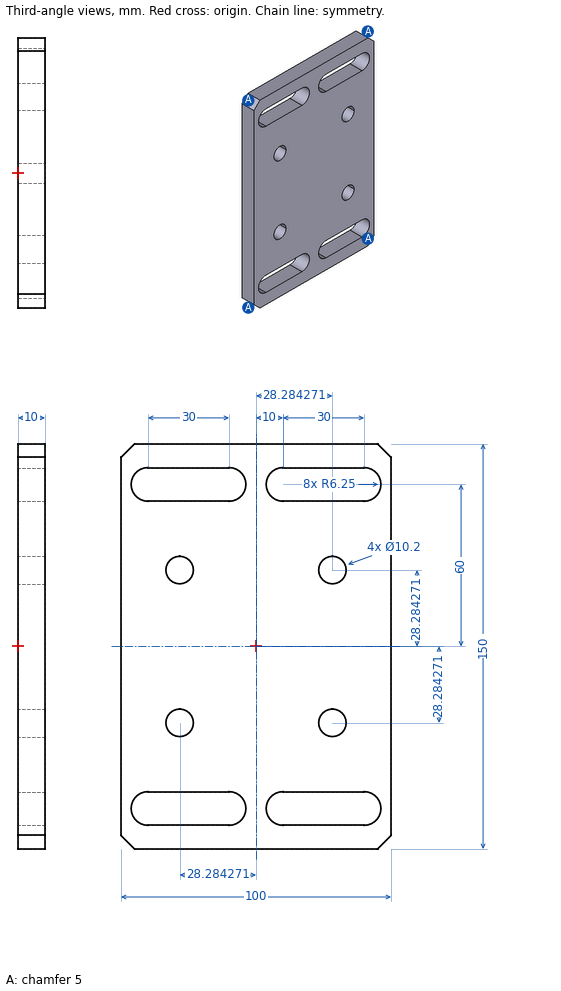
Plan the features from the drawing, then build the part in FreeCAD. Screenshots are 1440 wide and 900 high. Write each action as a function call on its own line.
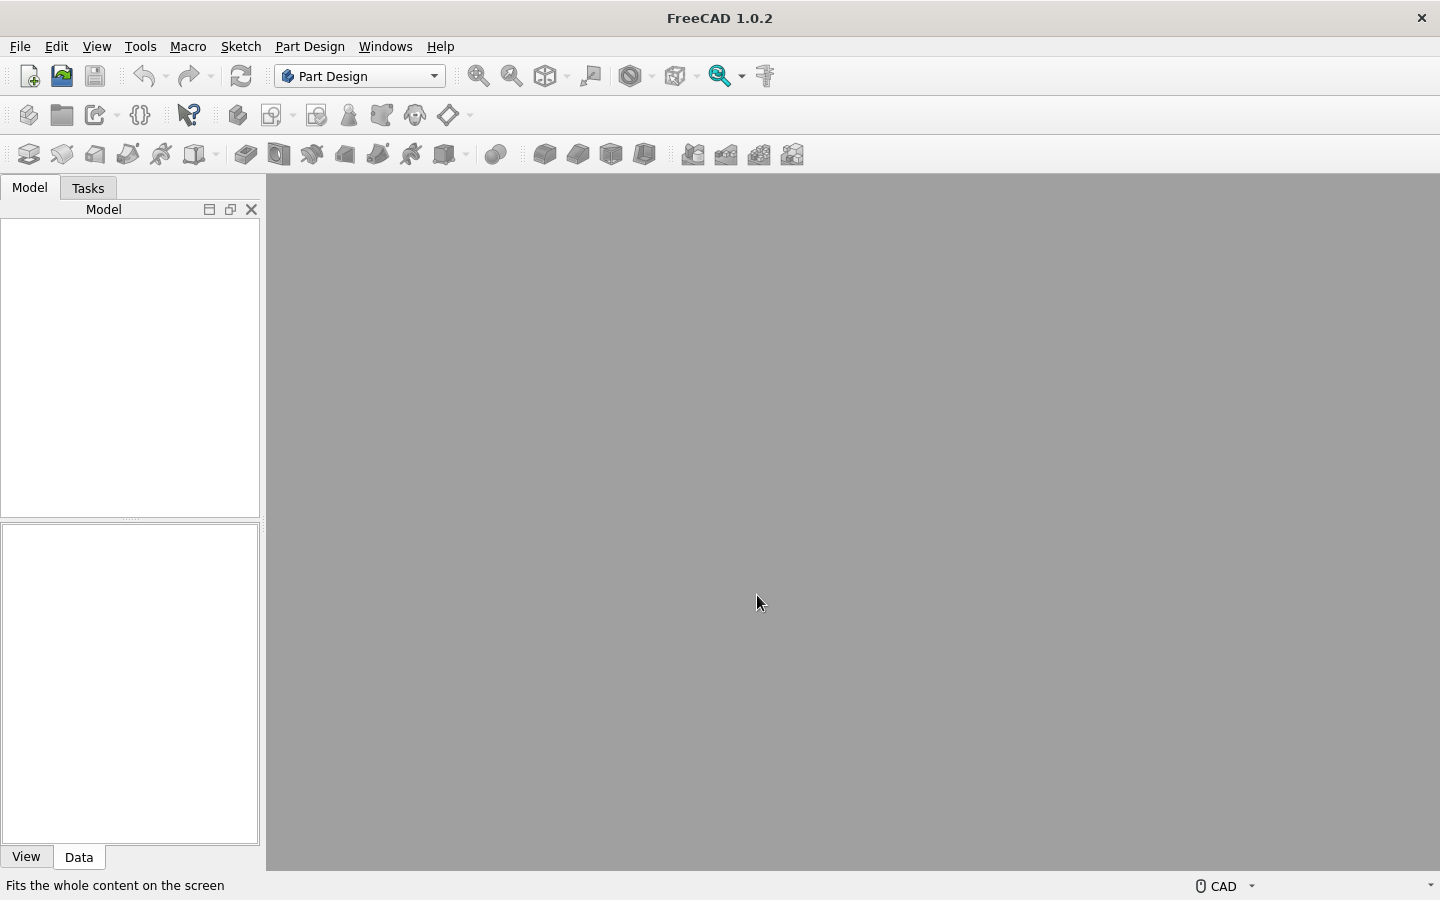
click(29, 76)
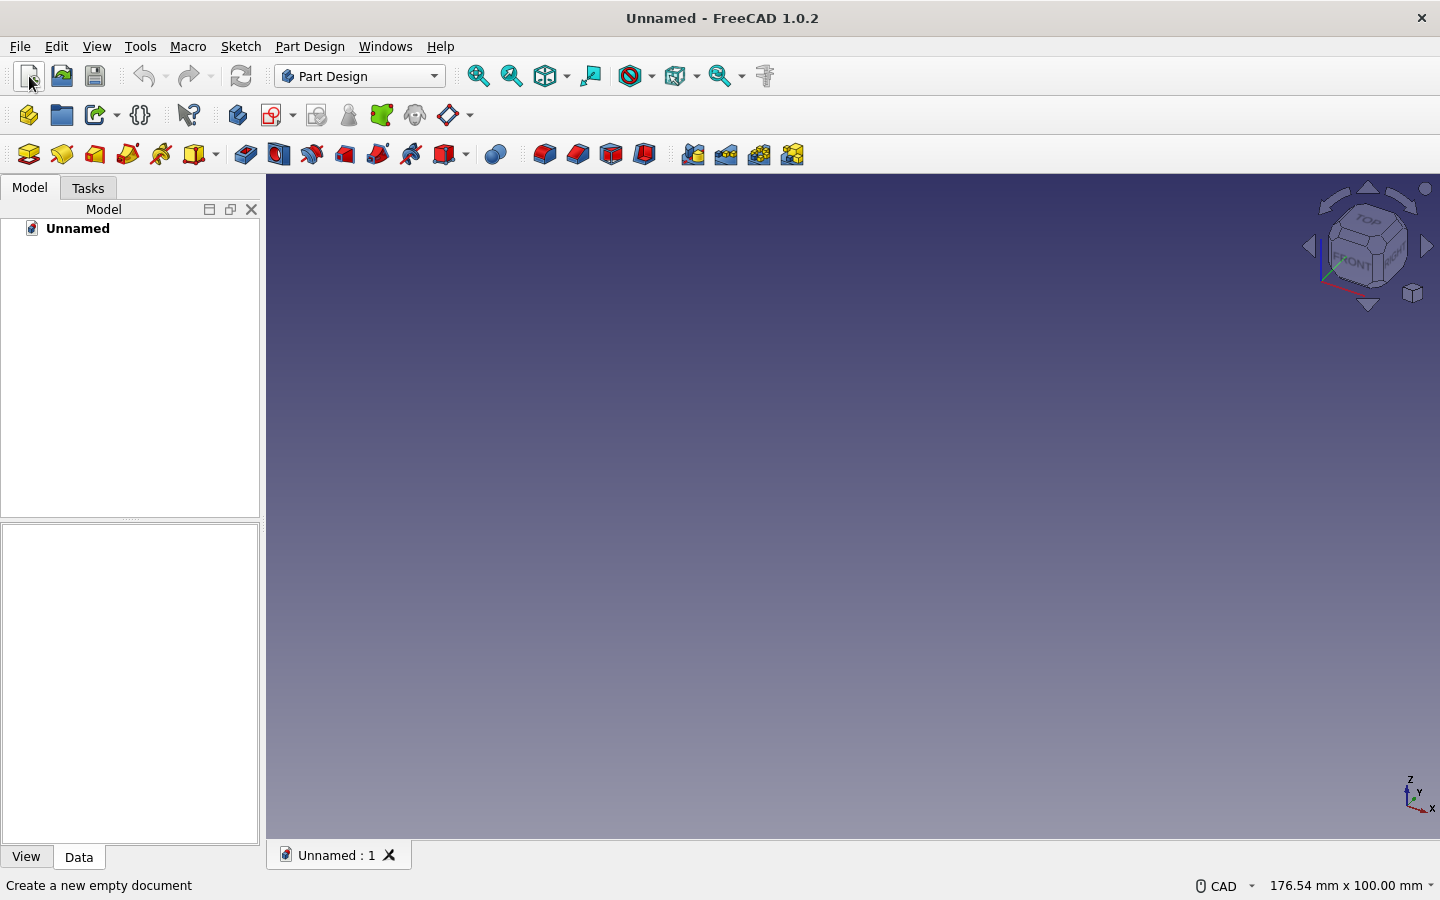
click(270, 116)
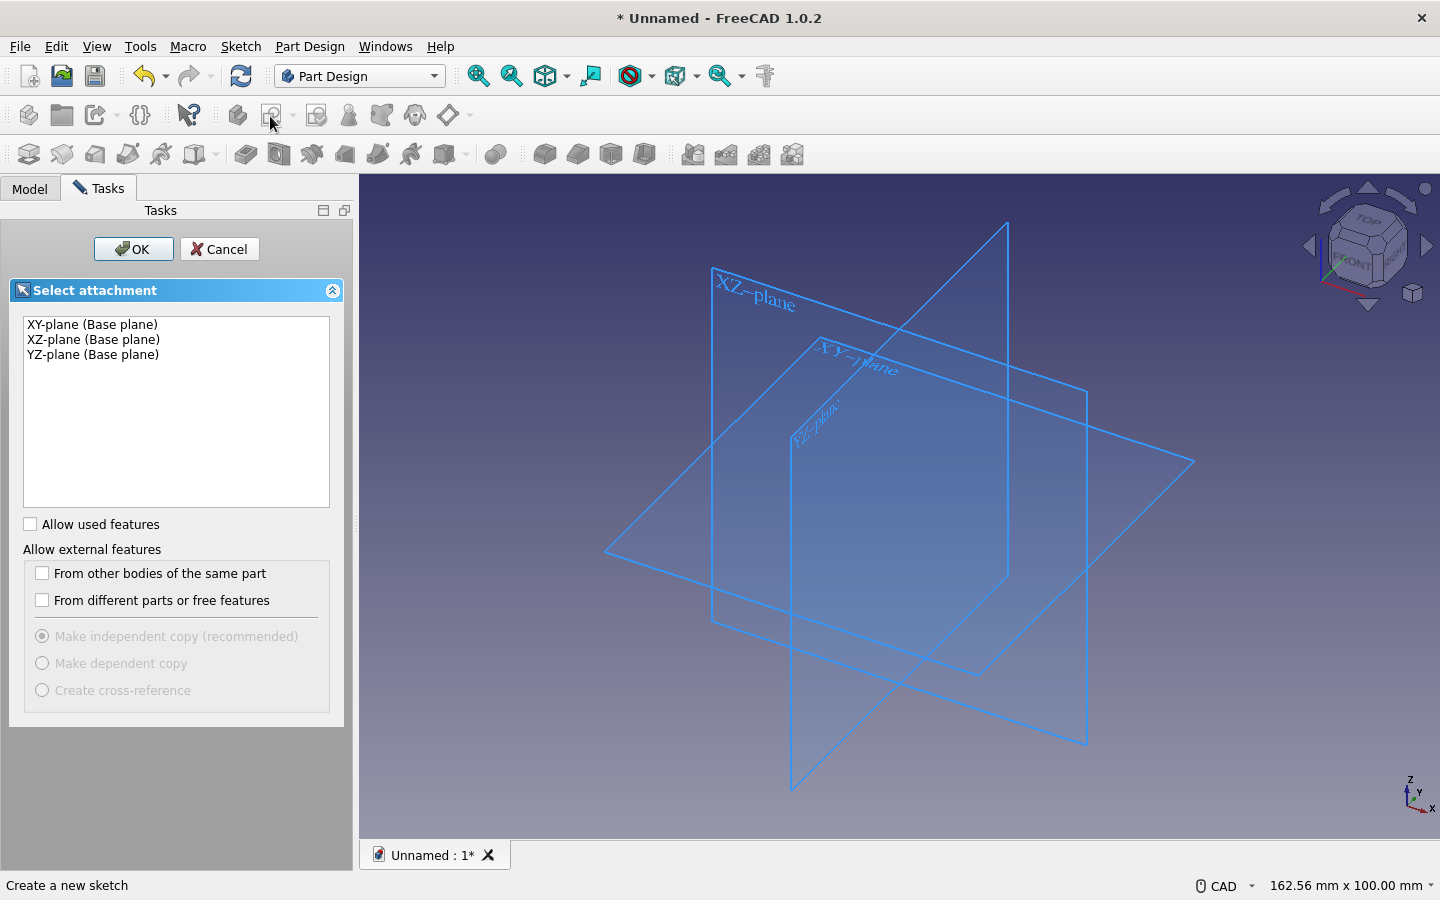
click(84, 354)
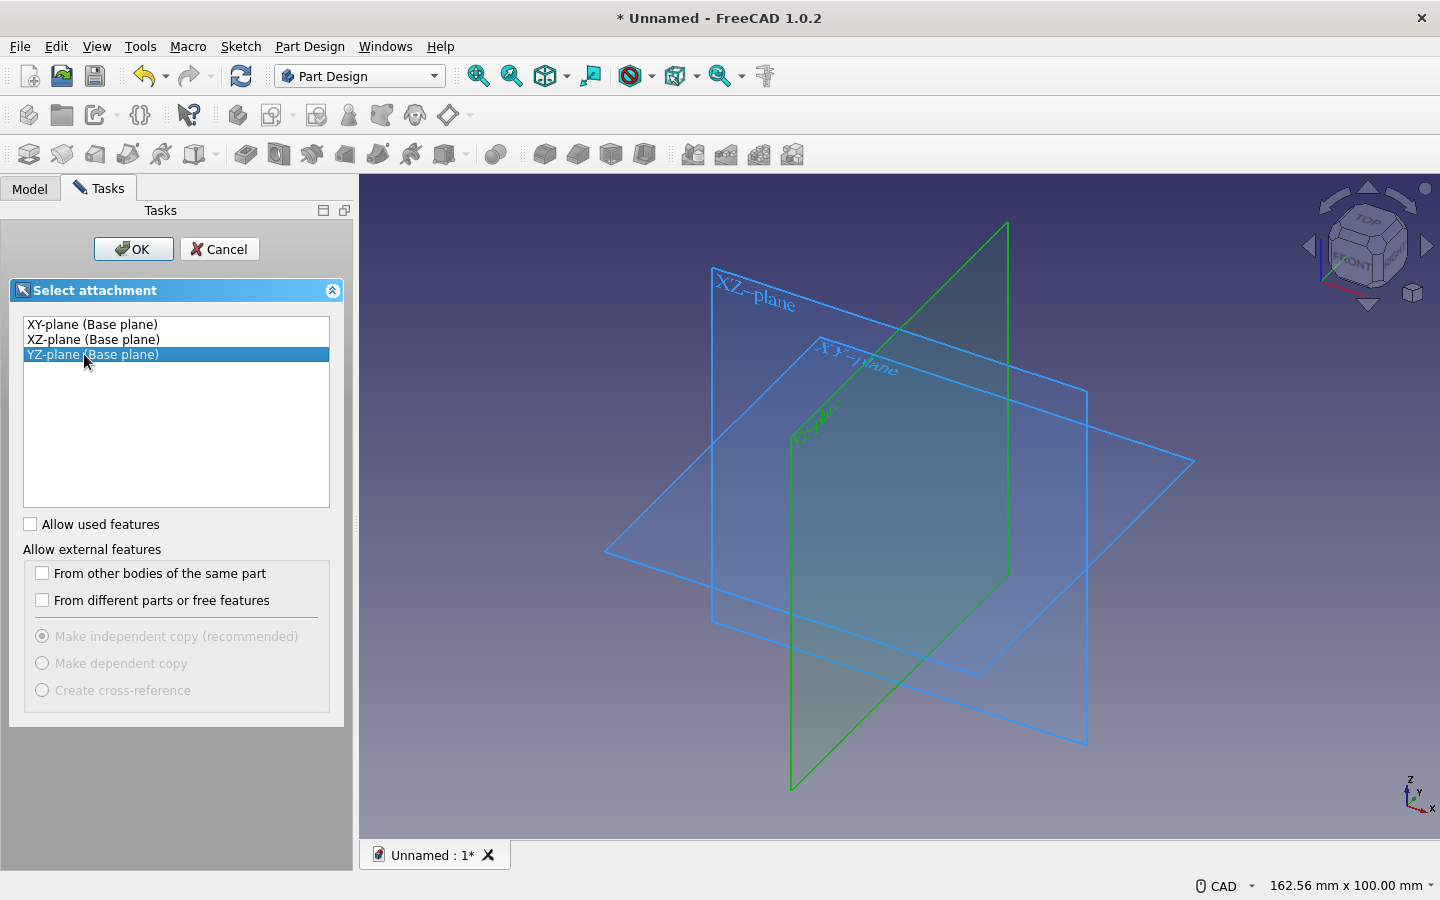
click(134, 249)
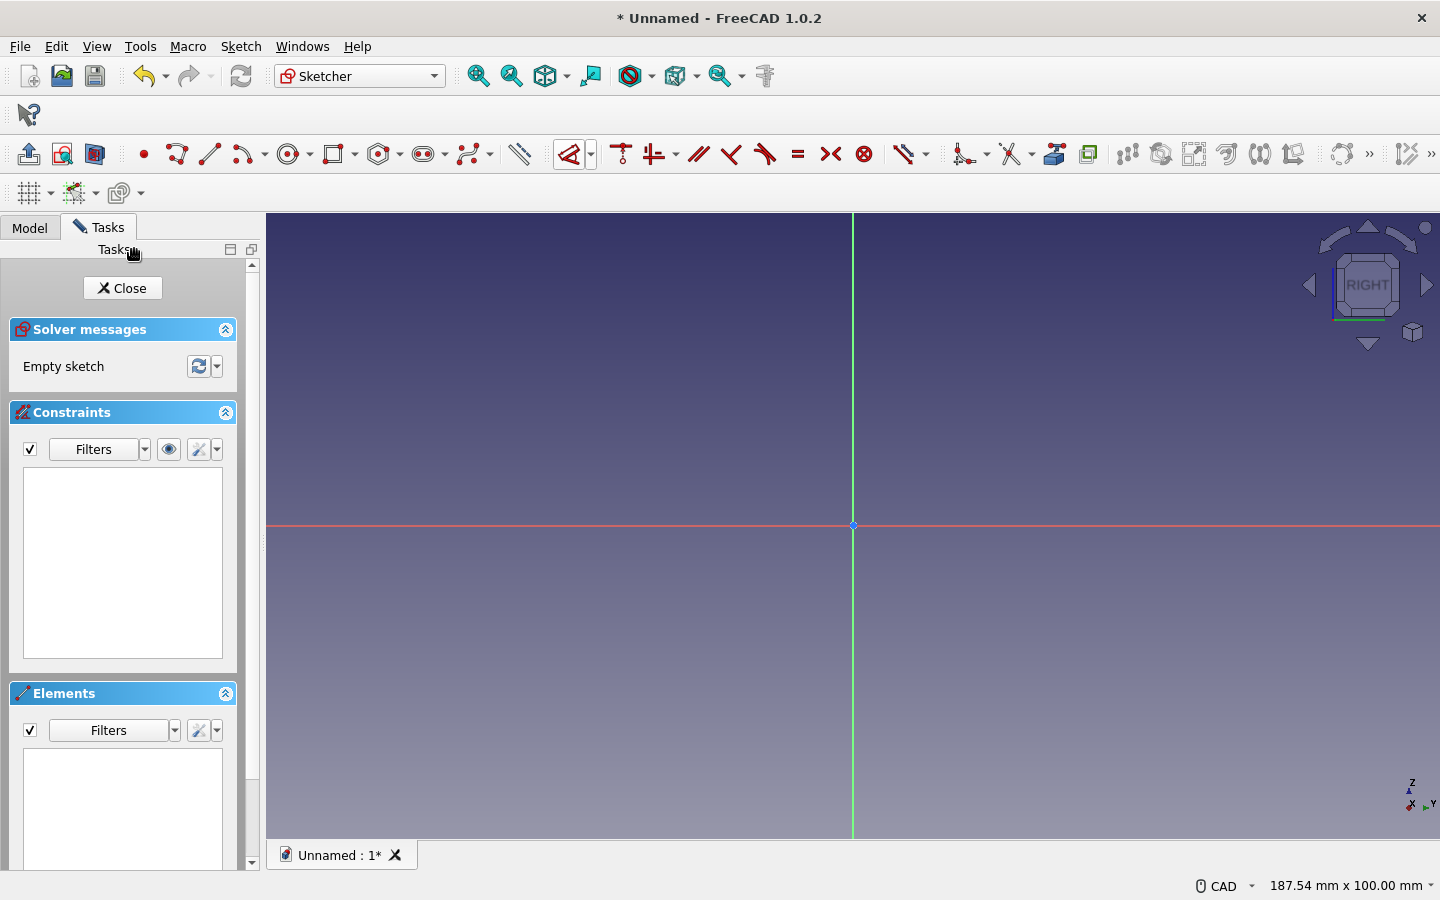
scroll(729, 526, down, 4)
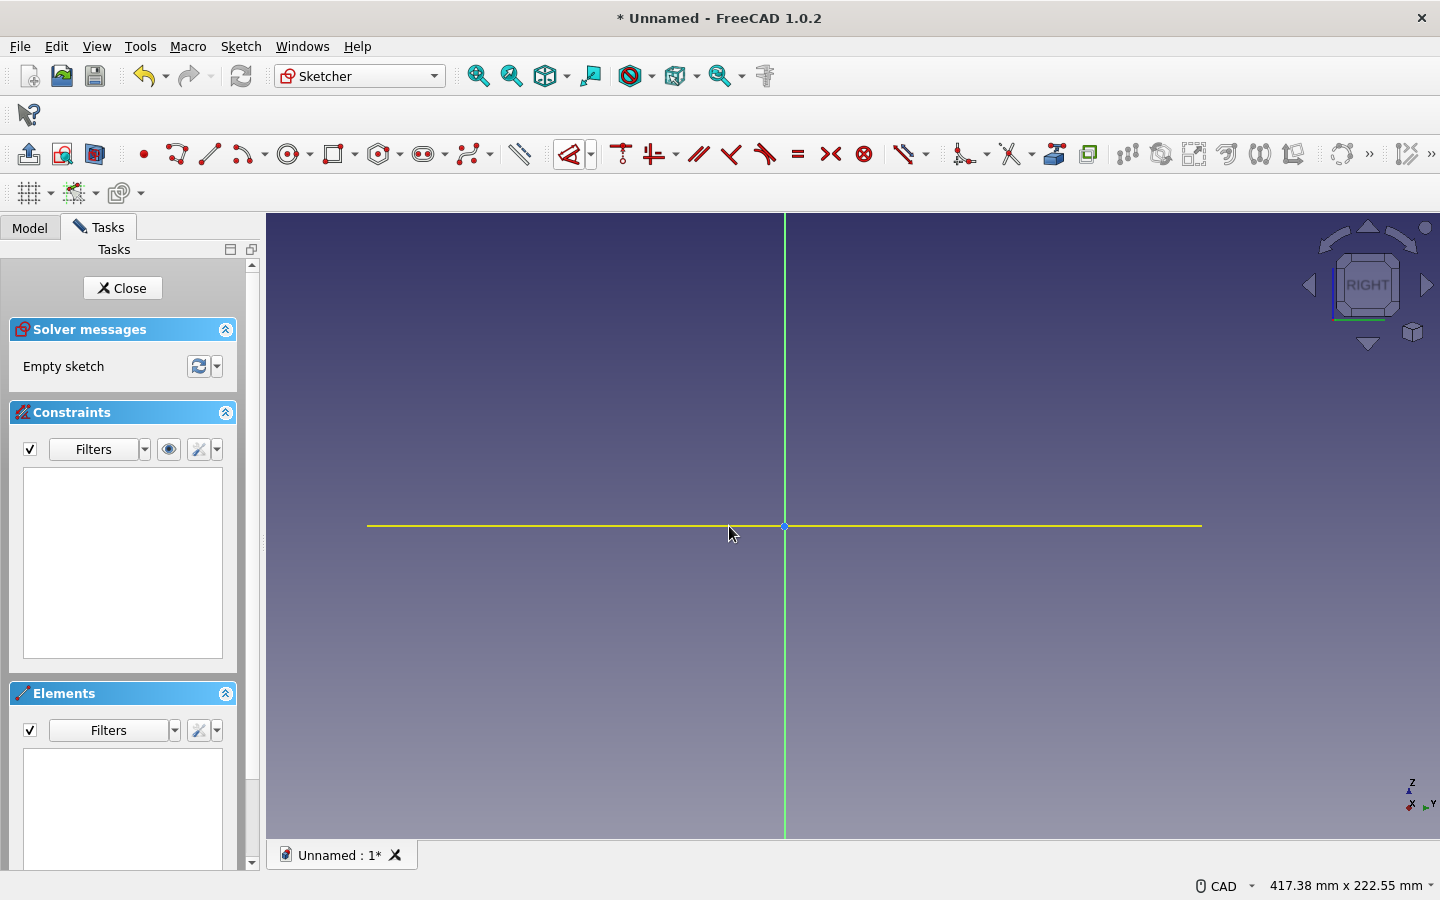
key(g)
key(v)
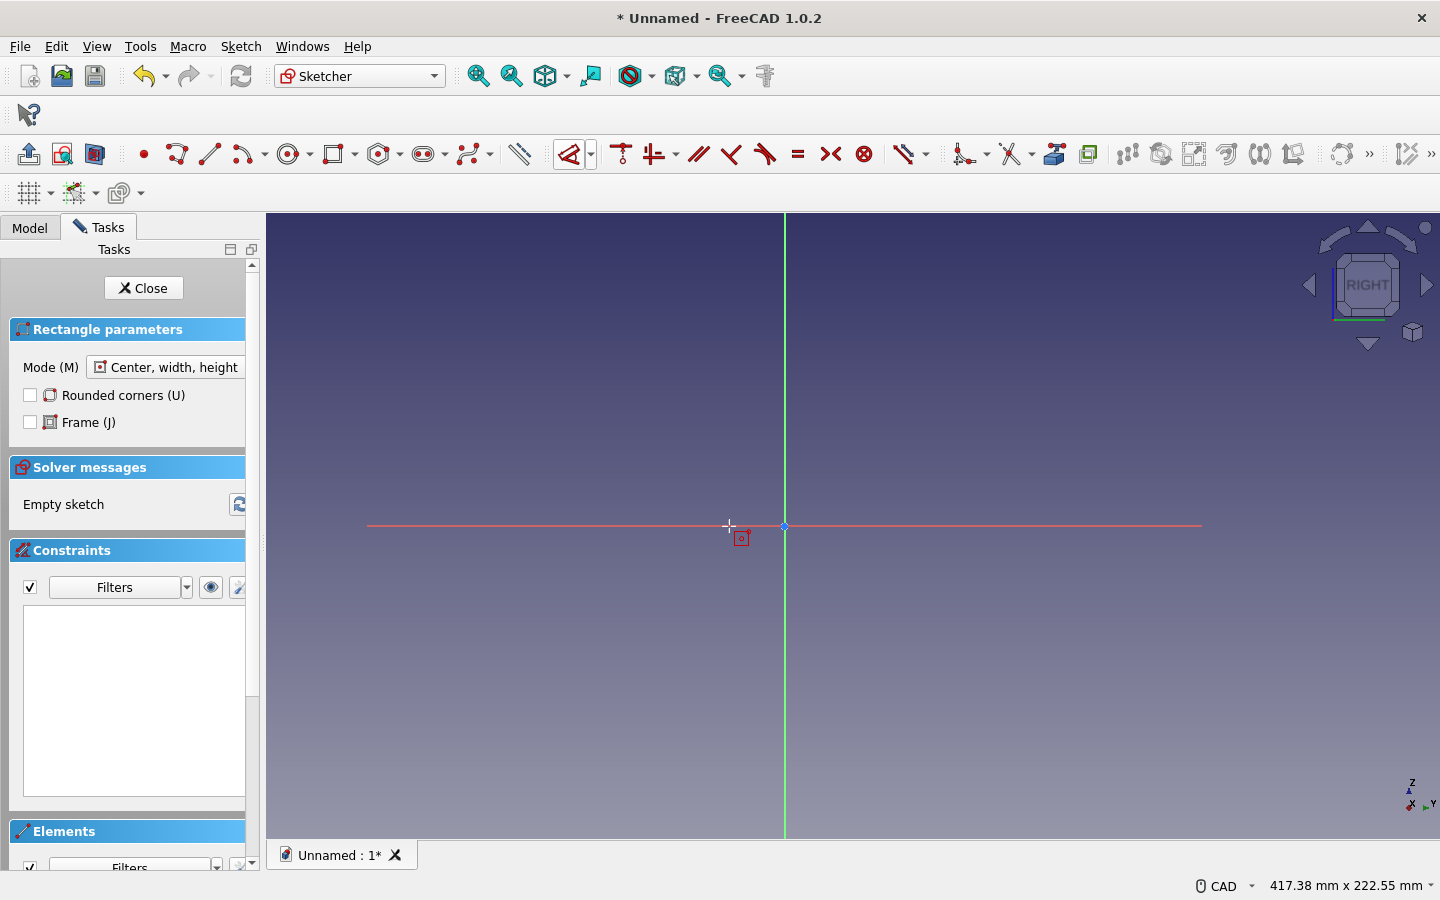
click(785, 526)
click(926, 315)
key(Escape)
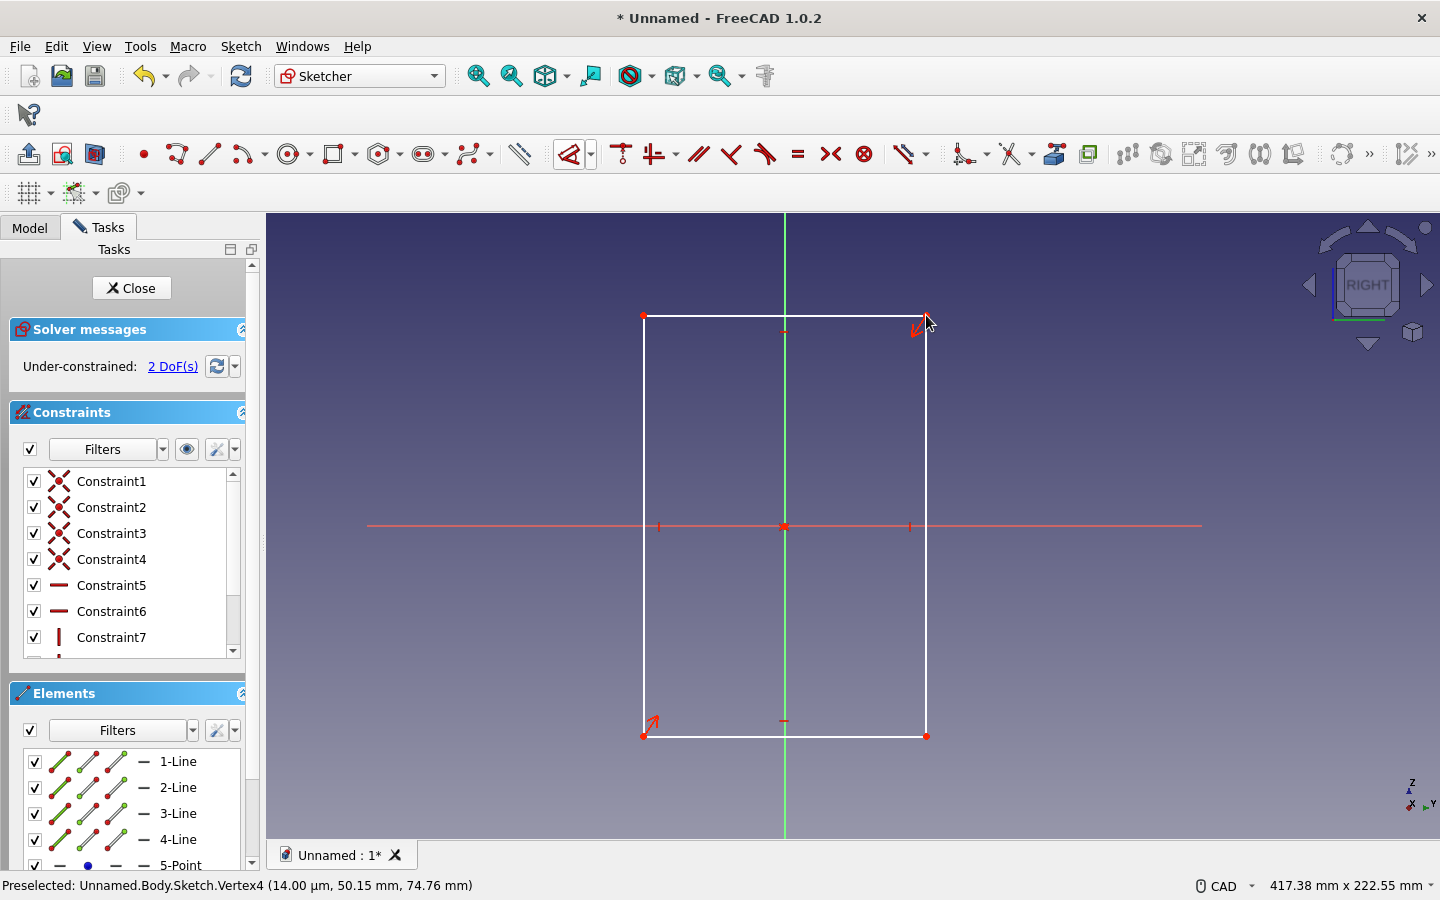
key(d)